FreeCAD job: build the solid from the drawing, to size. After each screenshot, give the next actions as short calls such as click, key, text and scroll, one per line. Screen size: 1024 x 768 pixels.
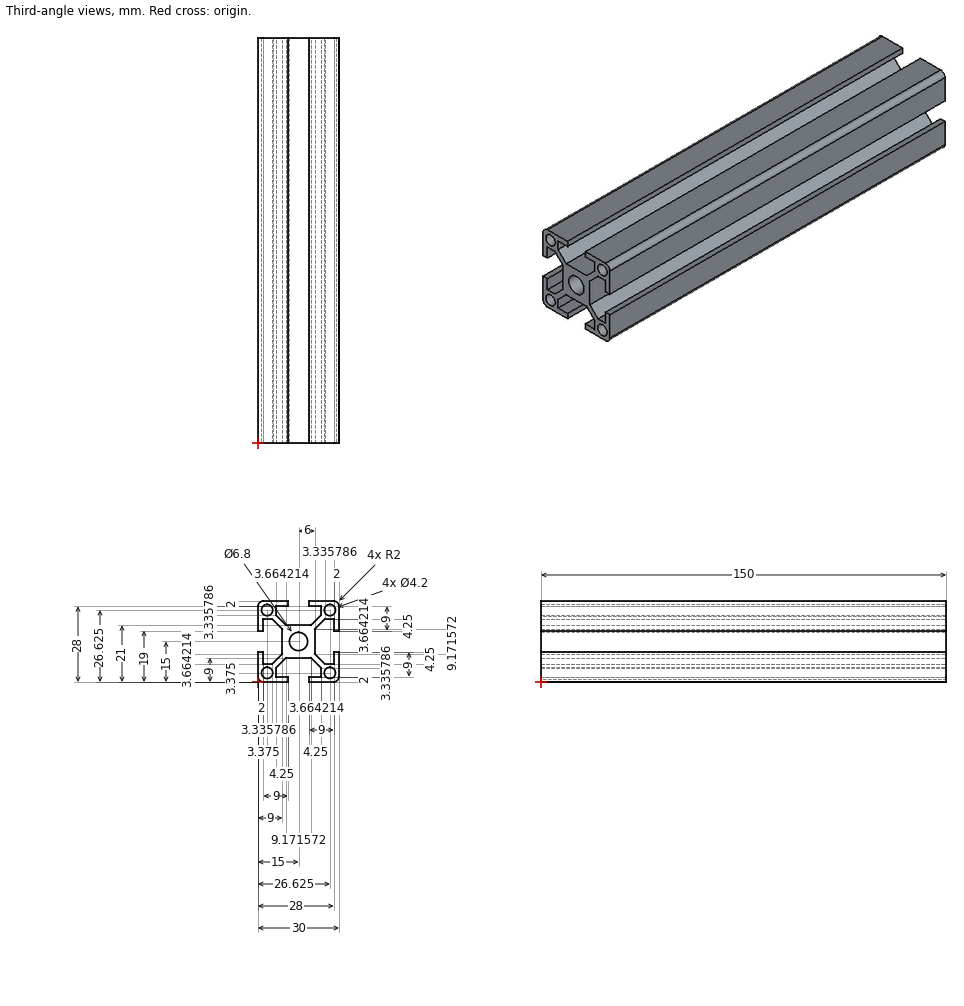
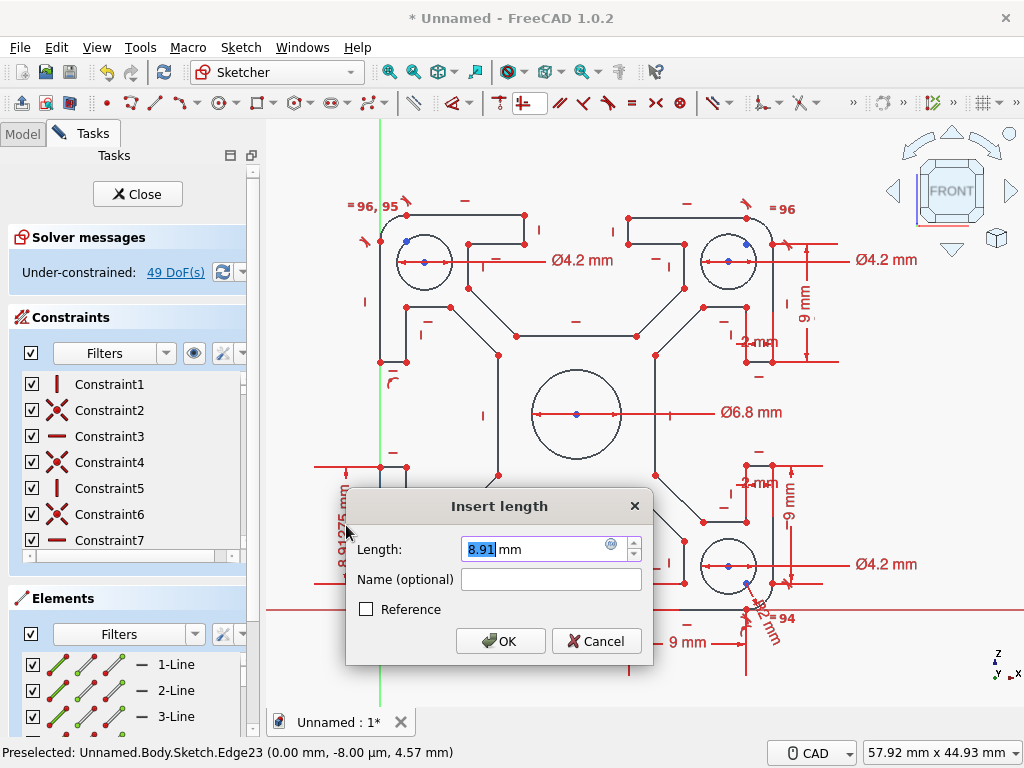
text(9)
key(Return)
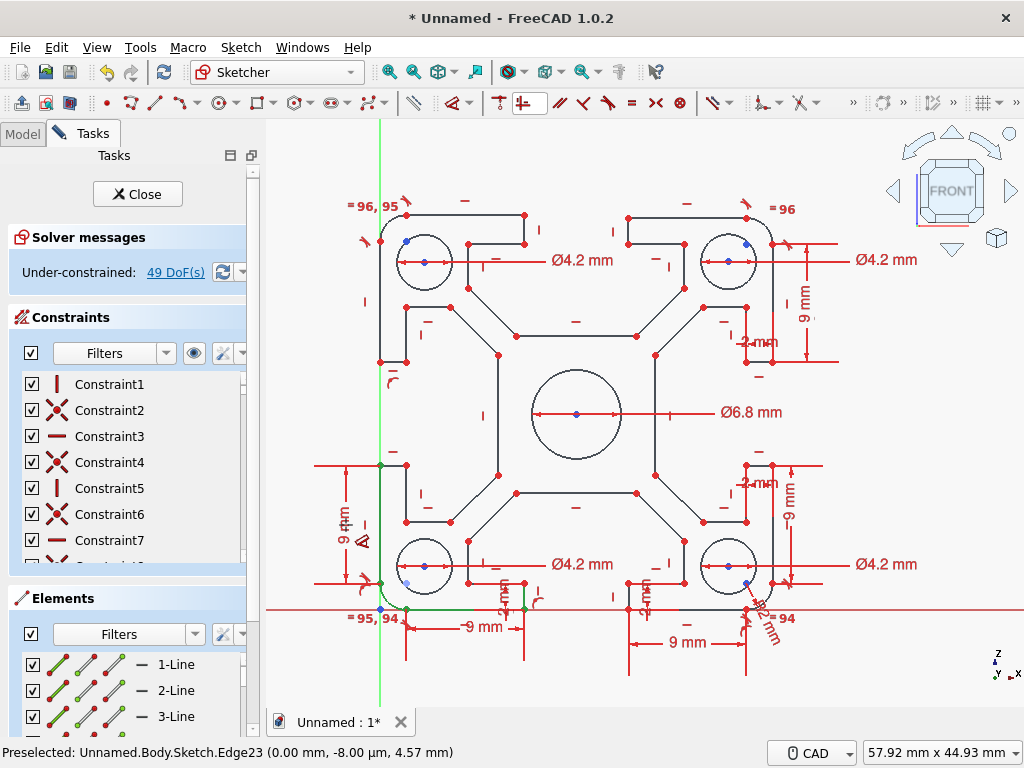
scroll(391, 466, up, 3)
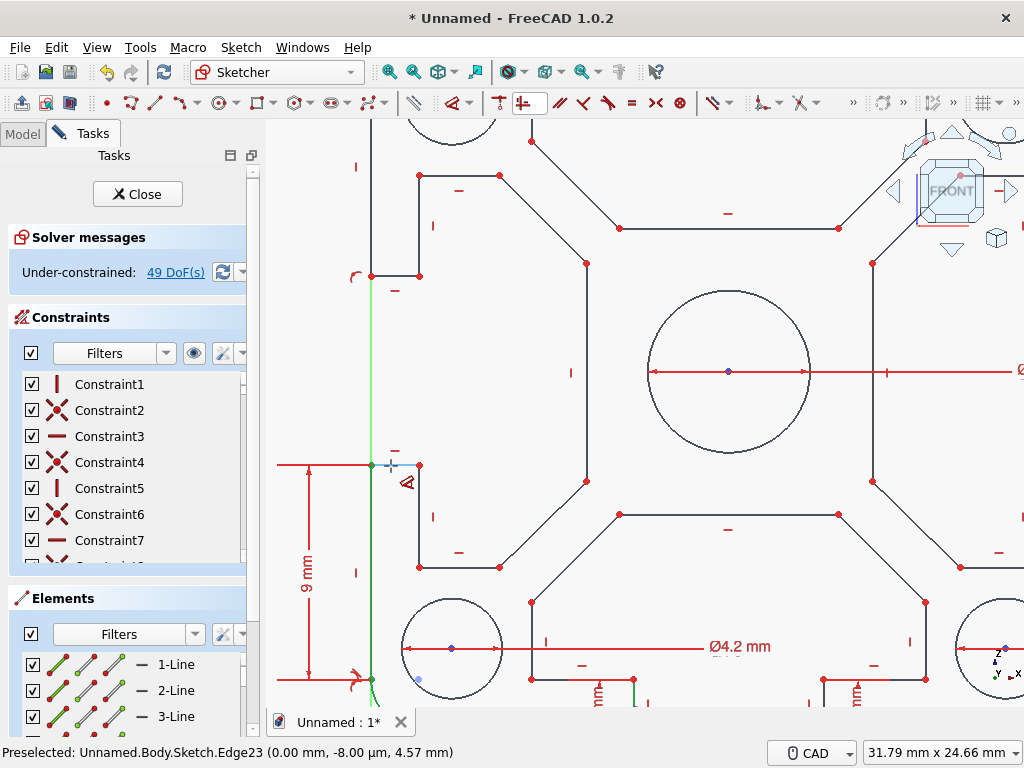
click(390, 465)
click(395, 499)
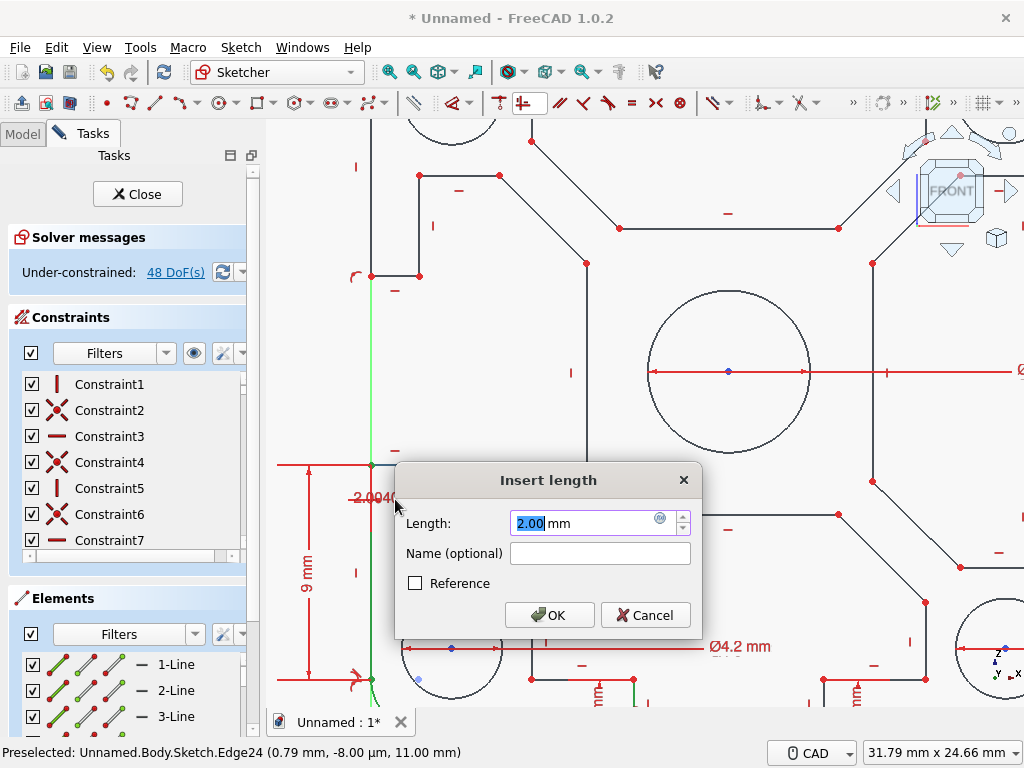
text(2)
key(Return)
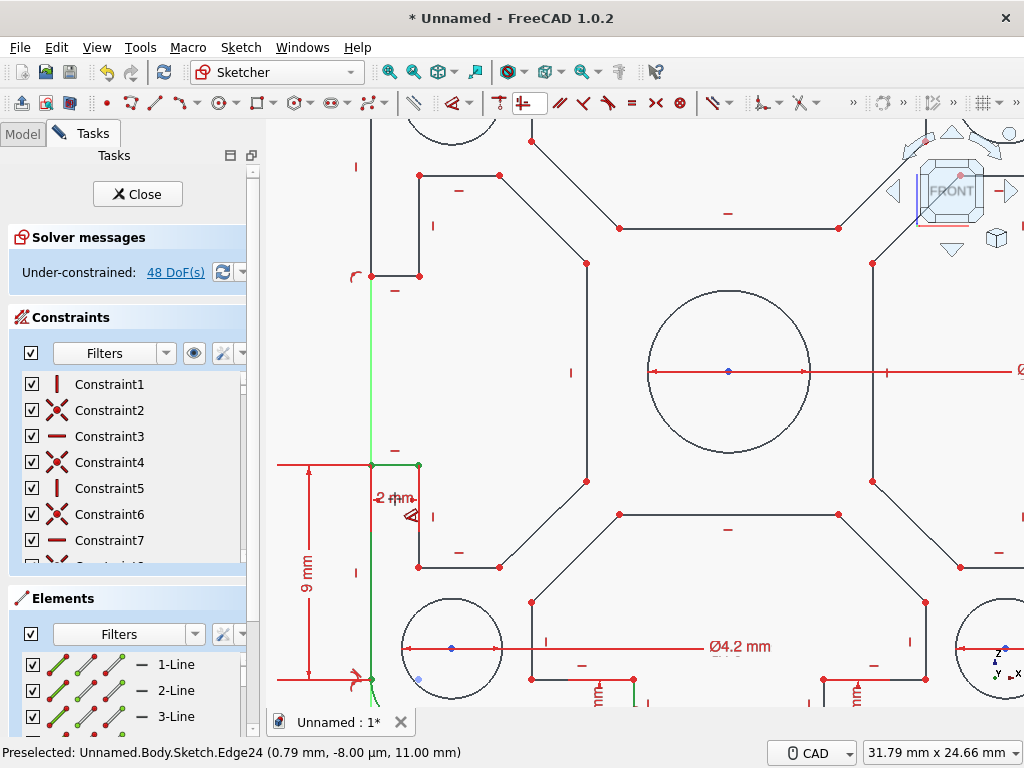
click(405, 276)
click(395, 242)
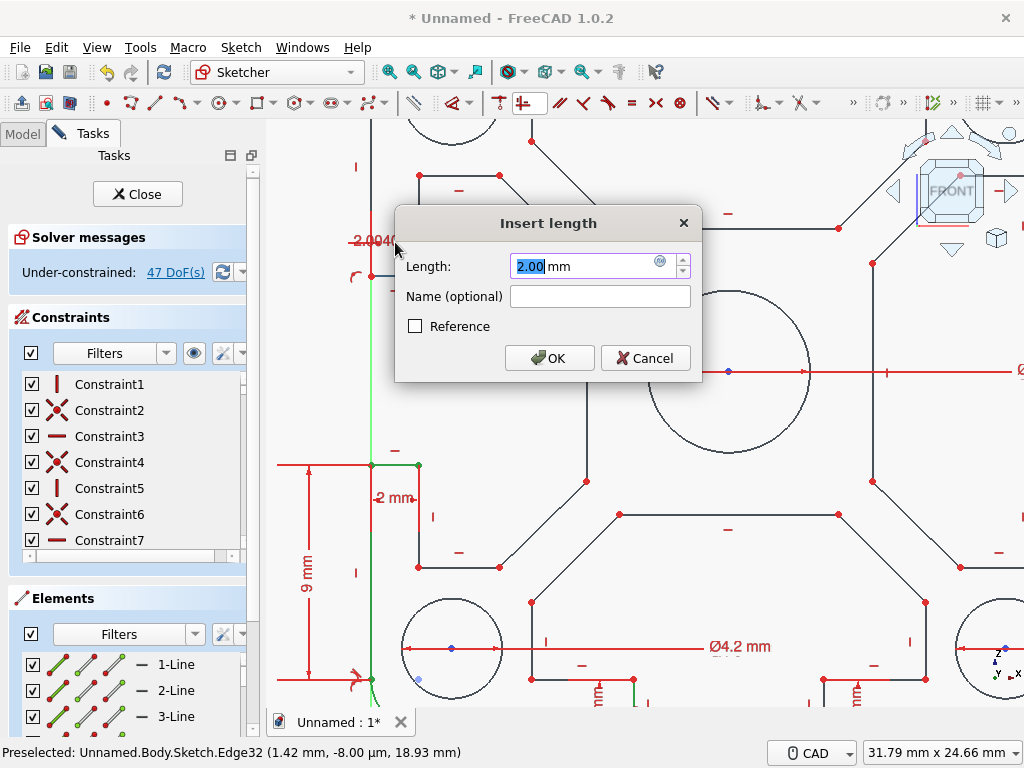
text(2)
key(Return)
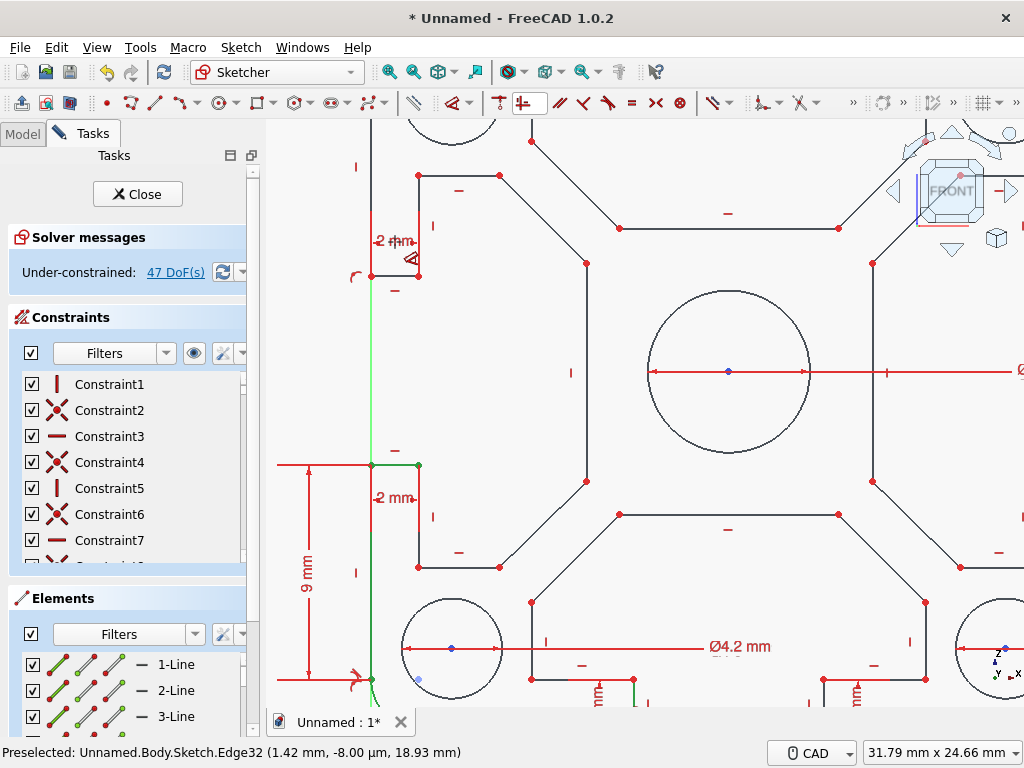
click(371, 210)
click(337, 212)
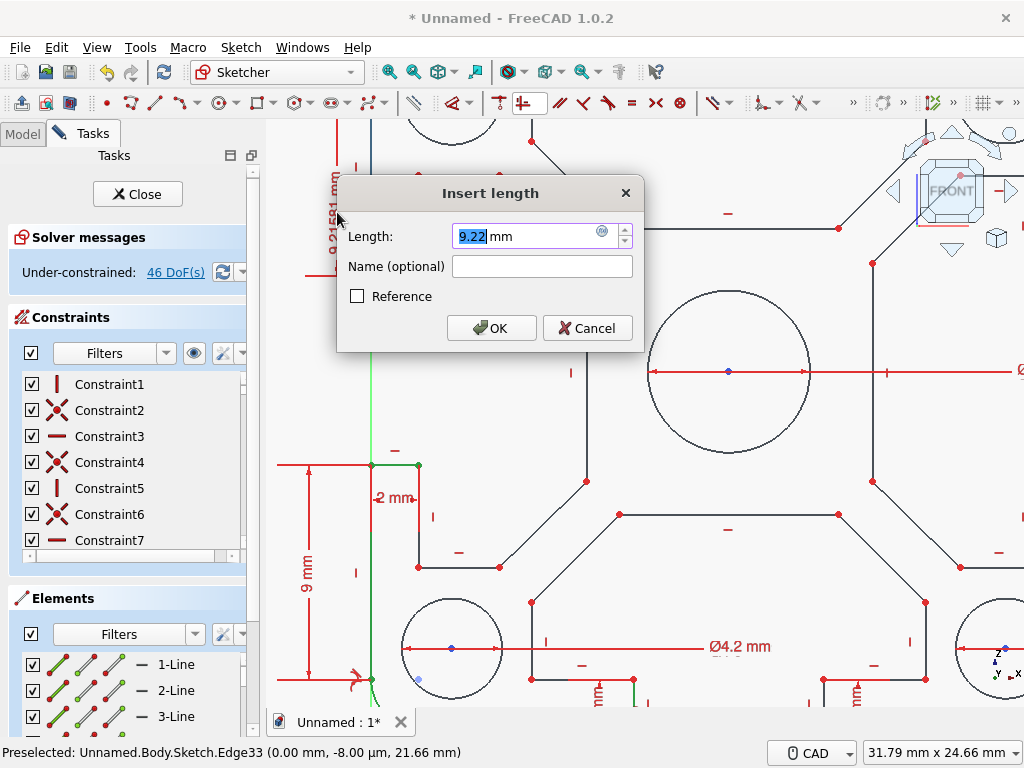
text(9)
key(Return)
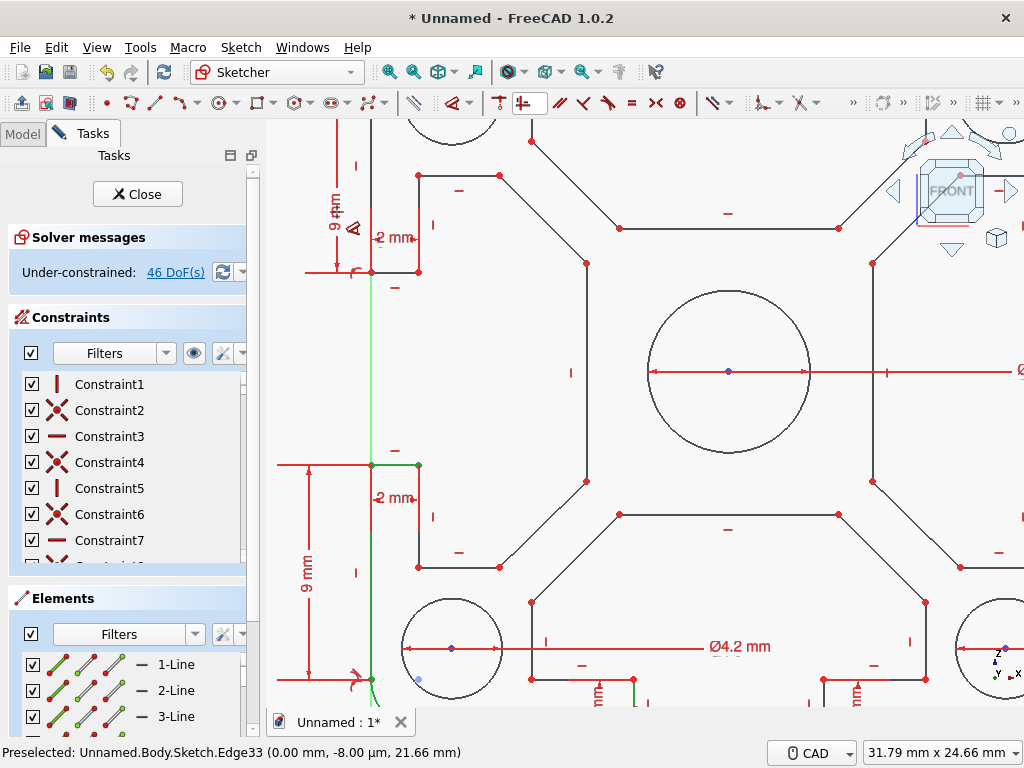
scroll(391, 465, down, 3)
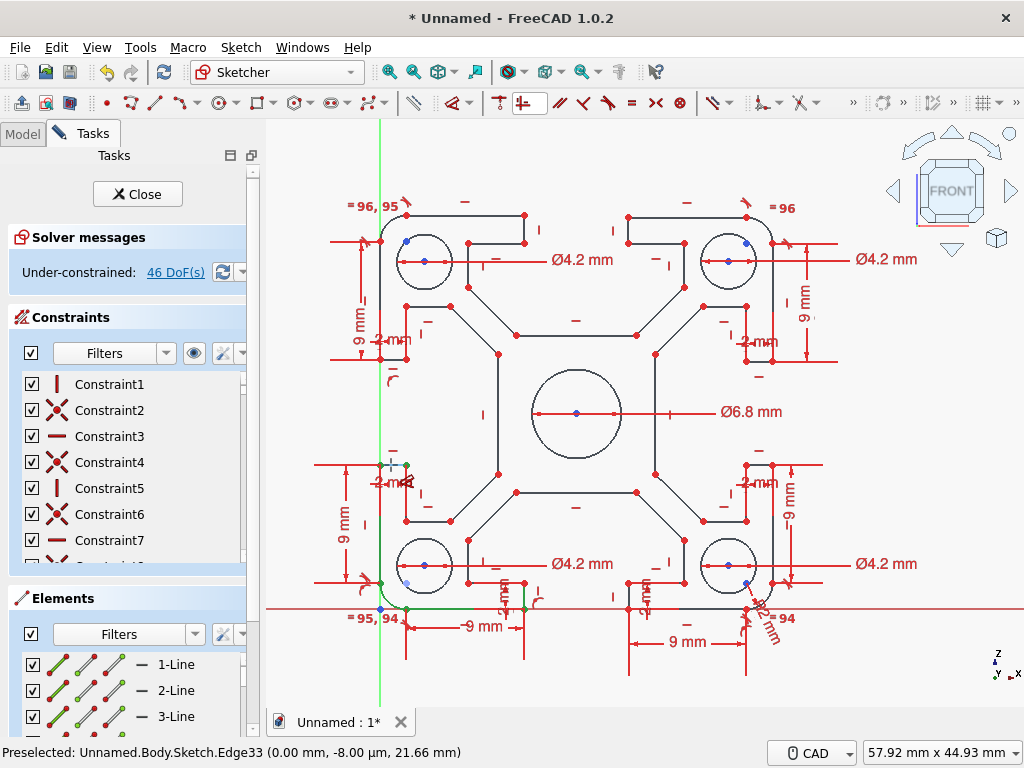
click(442, 216)
click(465, 182)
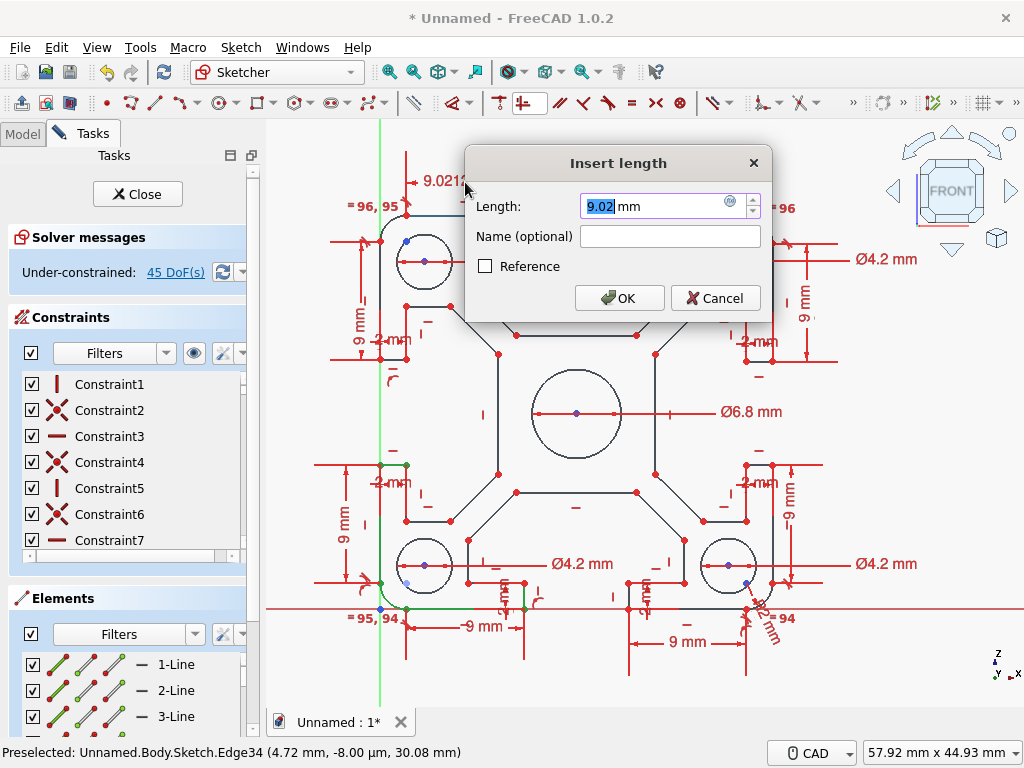
text(9)
key(Return)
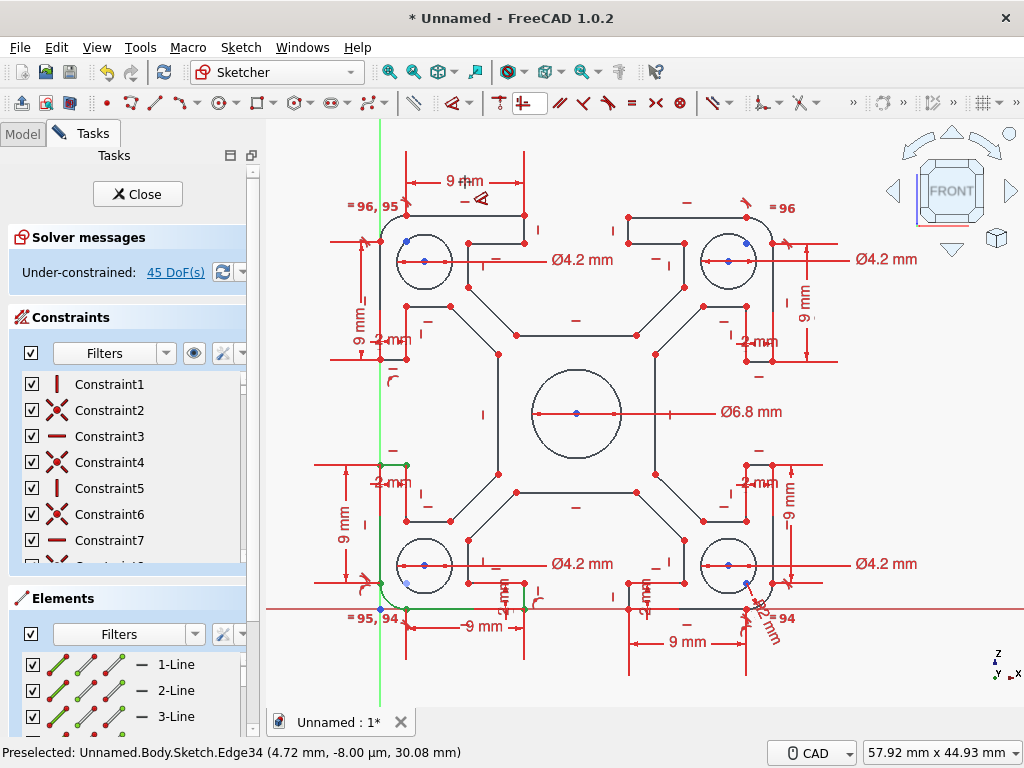
scroll(524, 227, up, 3)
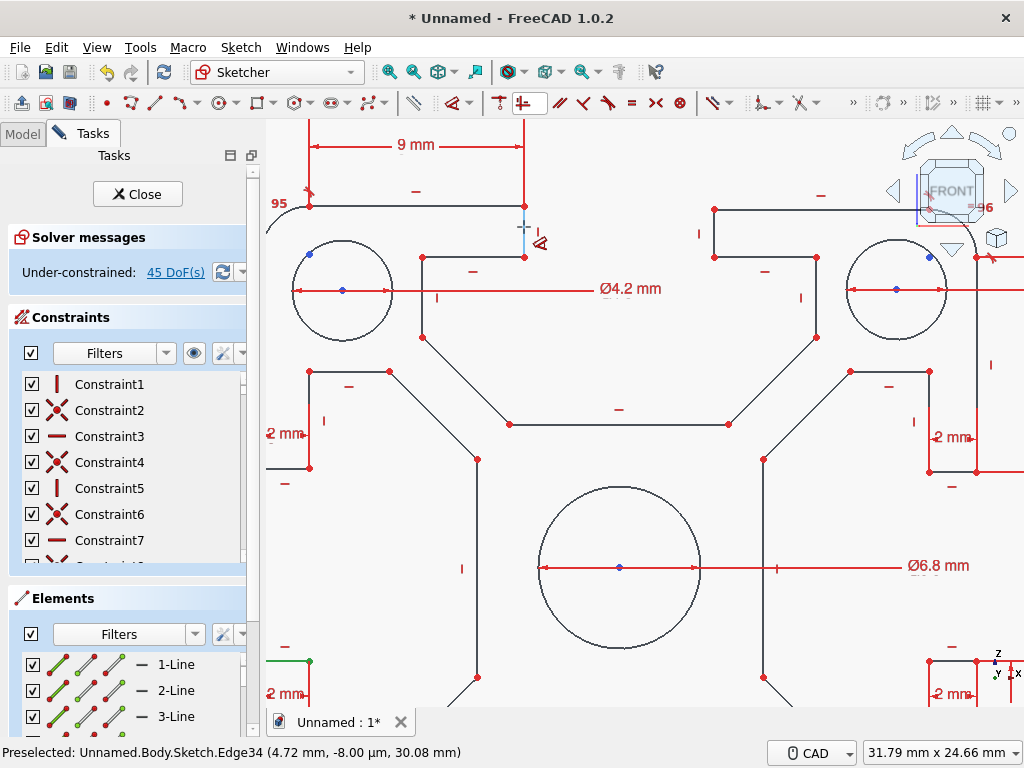
click(524, 227)
click(490, 232)